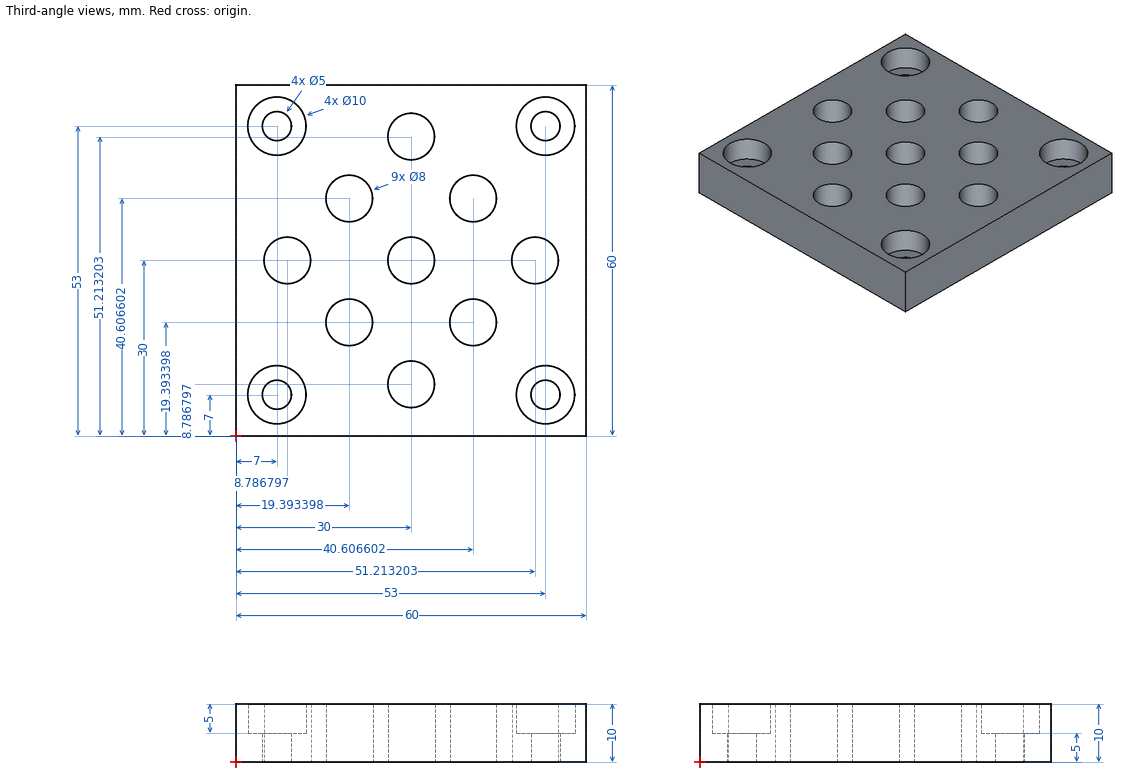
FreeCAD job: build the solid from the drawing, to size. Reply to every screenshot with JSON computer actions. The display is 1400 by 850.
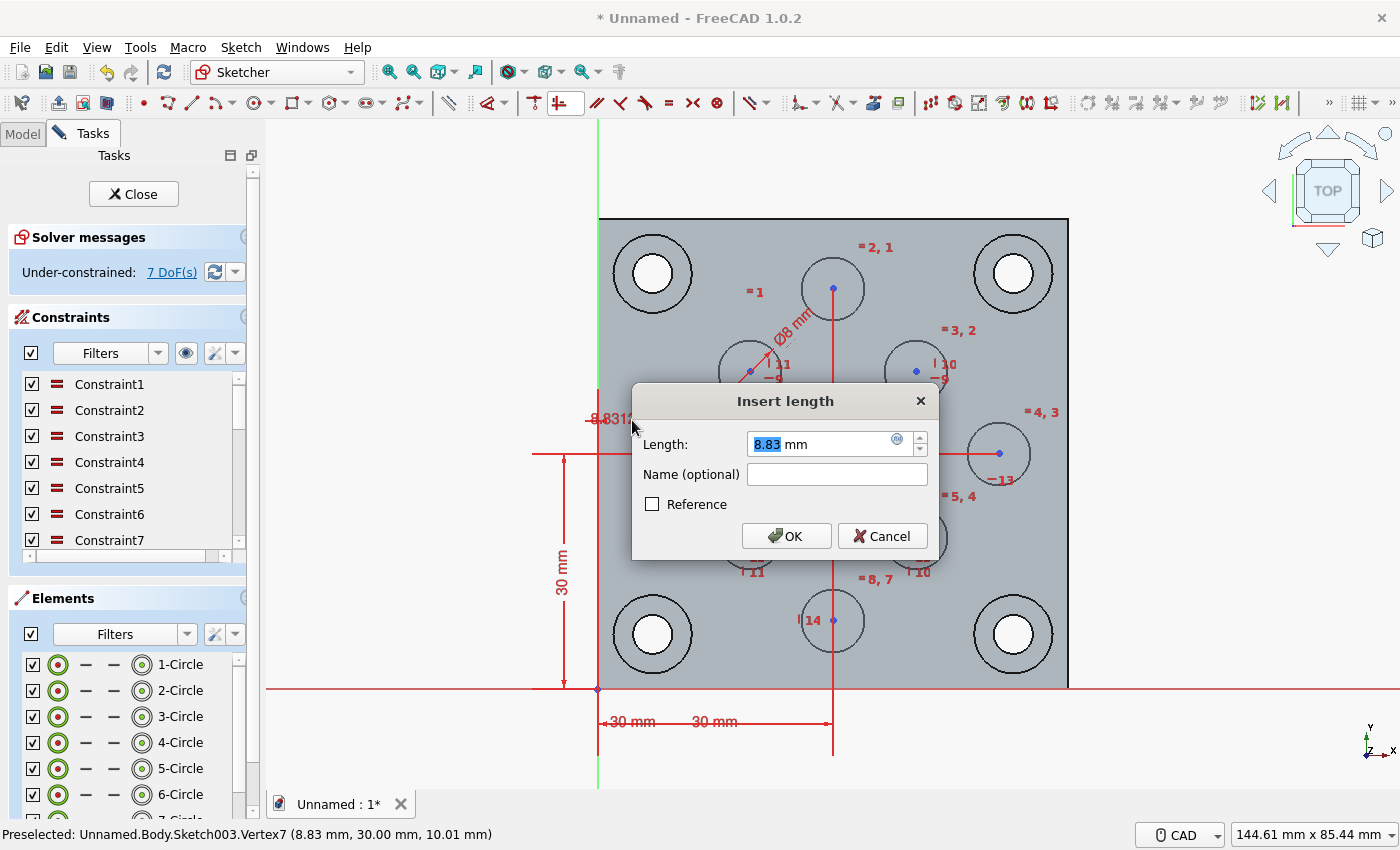
{"action": "type", "text": "8.786797"}
{"action": "key", "text": "Return"}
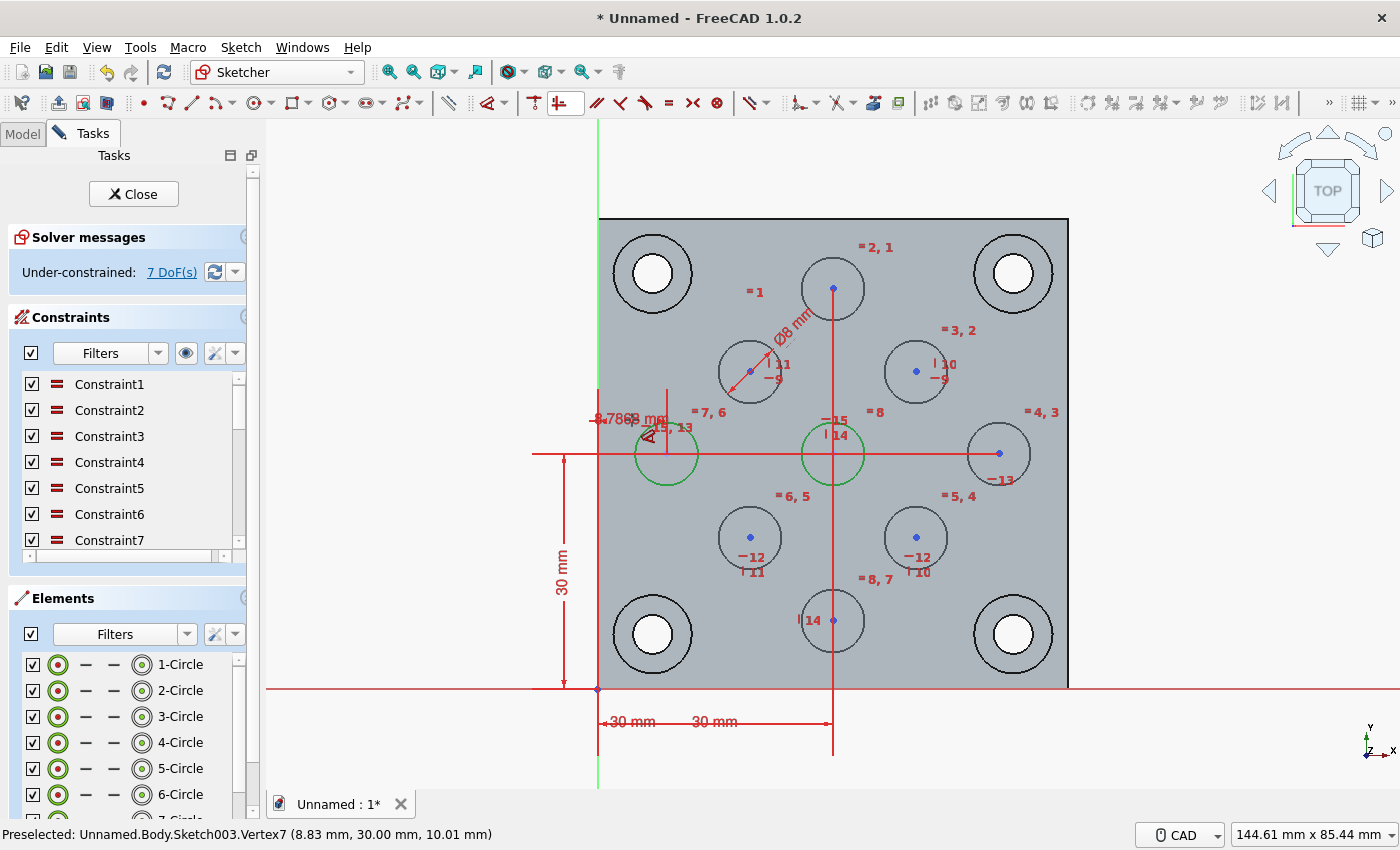
{"action": "left_click", "coordinate": [833, 621]}
{"action": "left_click", "coordinate": [564, 655]}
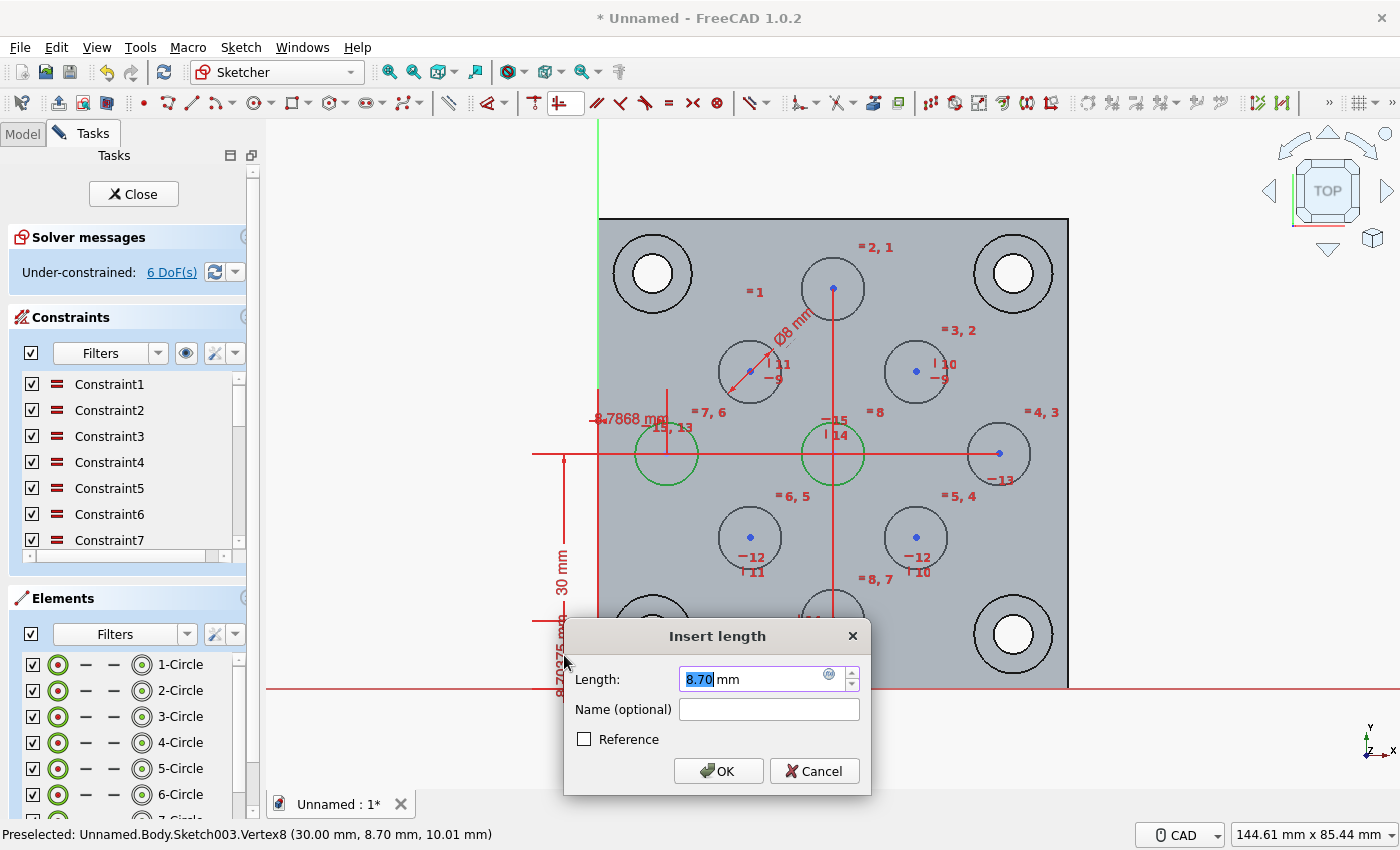
{"action": "type", "text": "8.786797"}
{"action": "key", "text": "Return"}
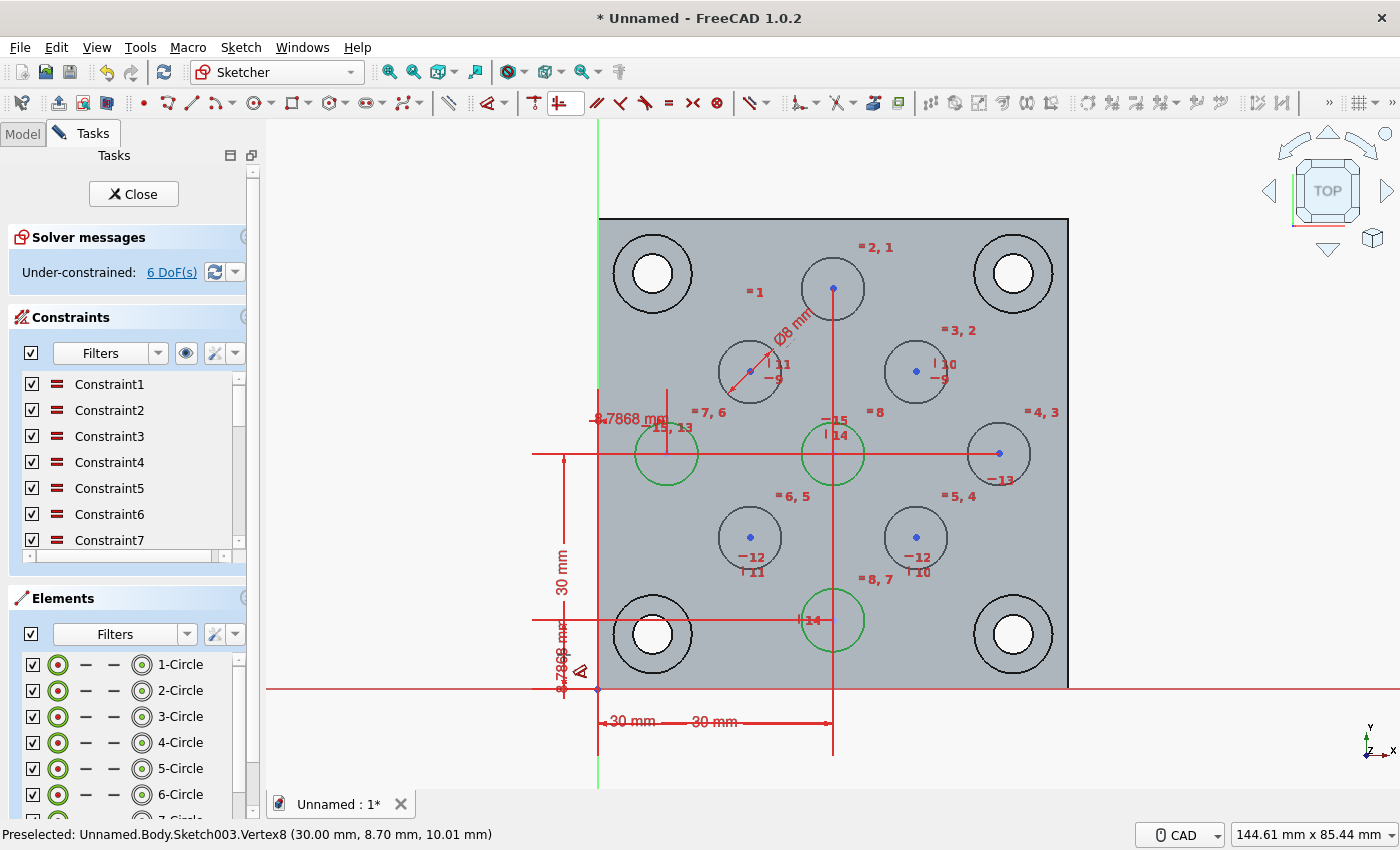
{"action": "left_click", "coordinate": [750, 372]}
{"action": "left_click", "coordinate": [674, 338]}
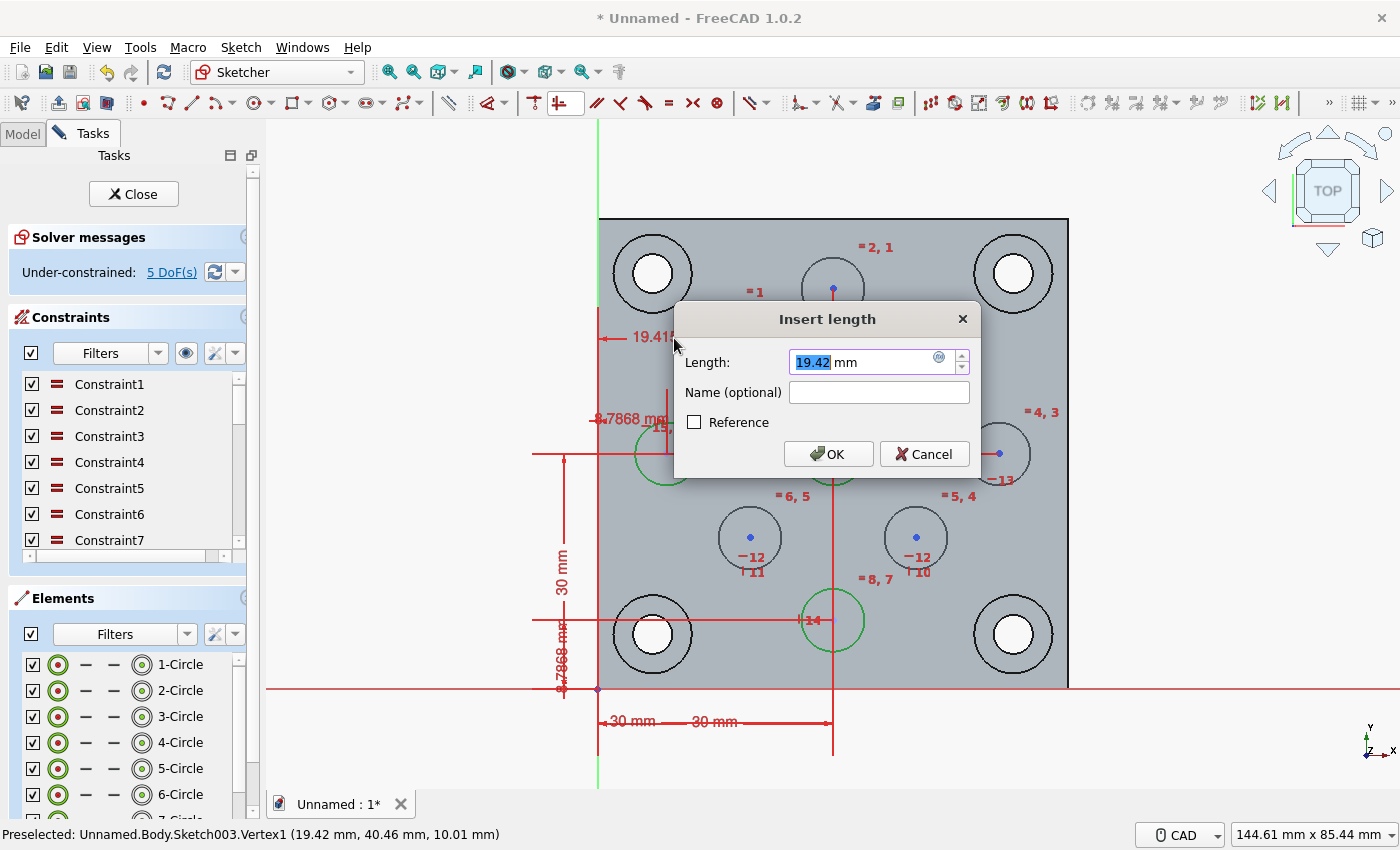
{"action": "type", "text": "19.393398"}
{"action": "key", "text": "Return"}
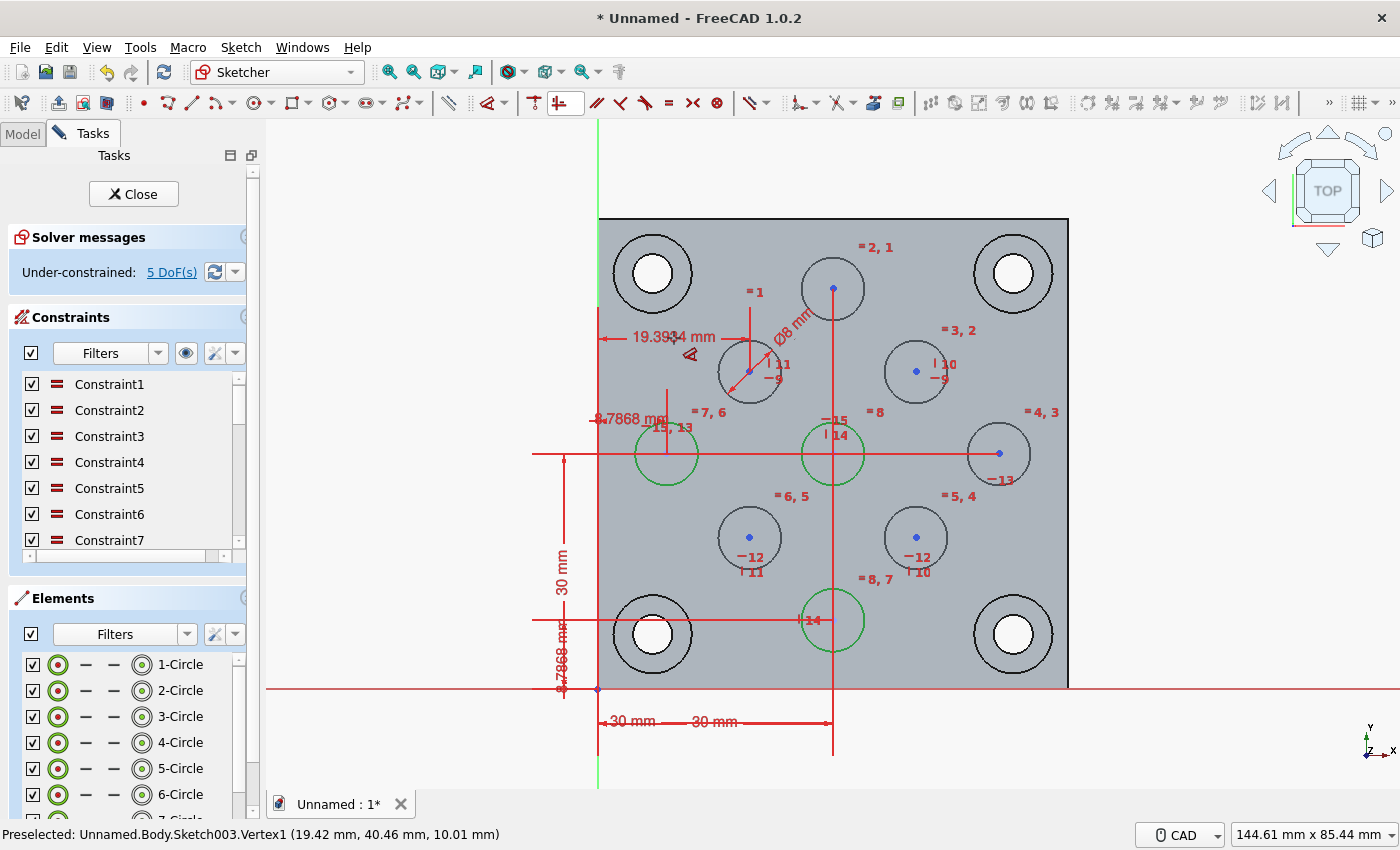
{"action": "left_click", "coordinate": [750, 372]}
{"action": "left_click", "coordinate": [564, 531]}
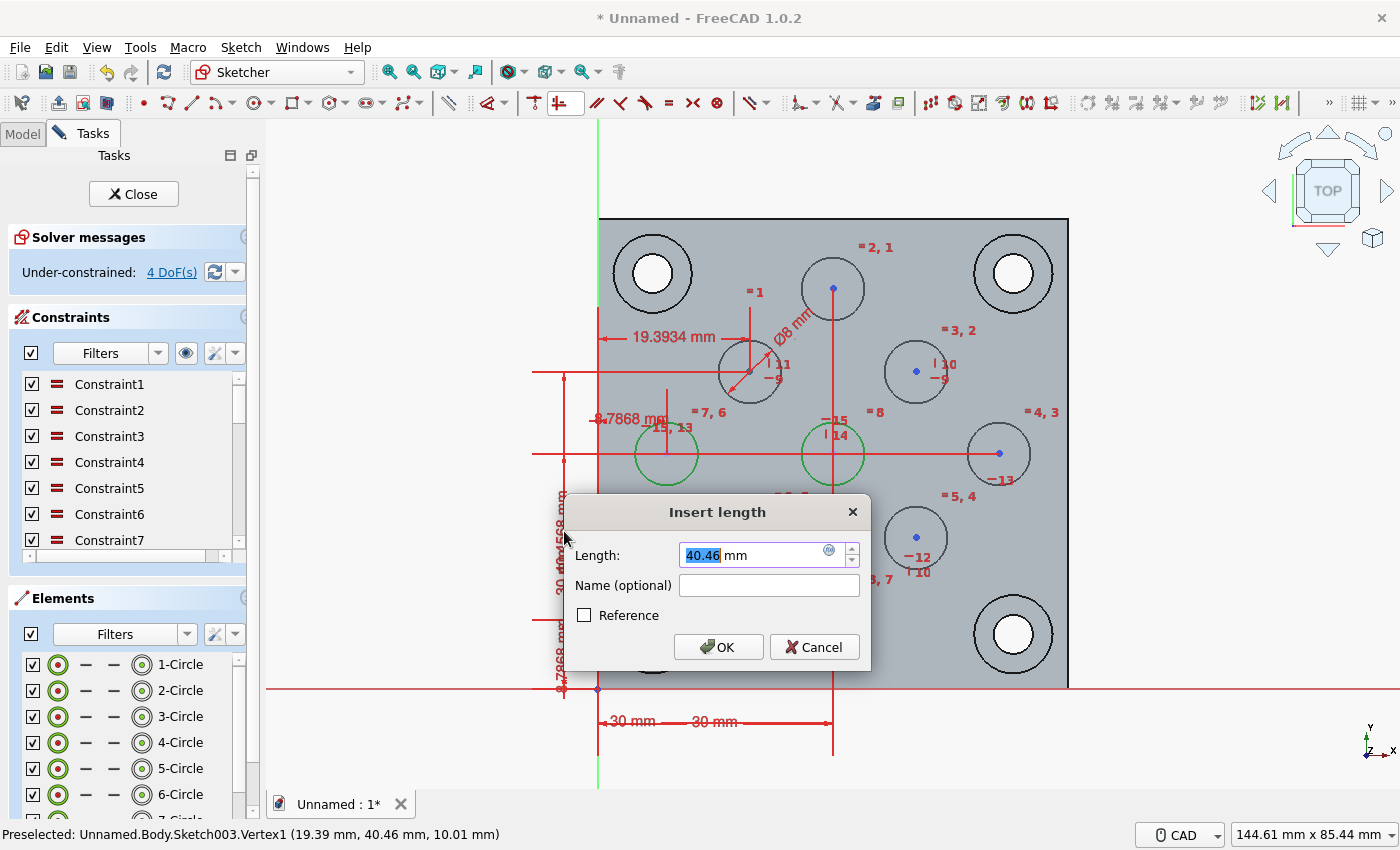
{"action": "type", "text": "40.606602"}
{"action": "key", "text": "Return"}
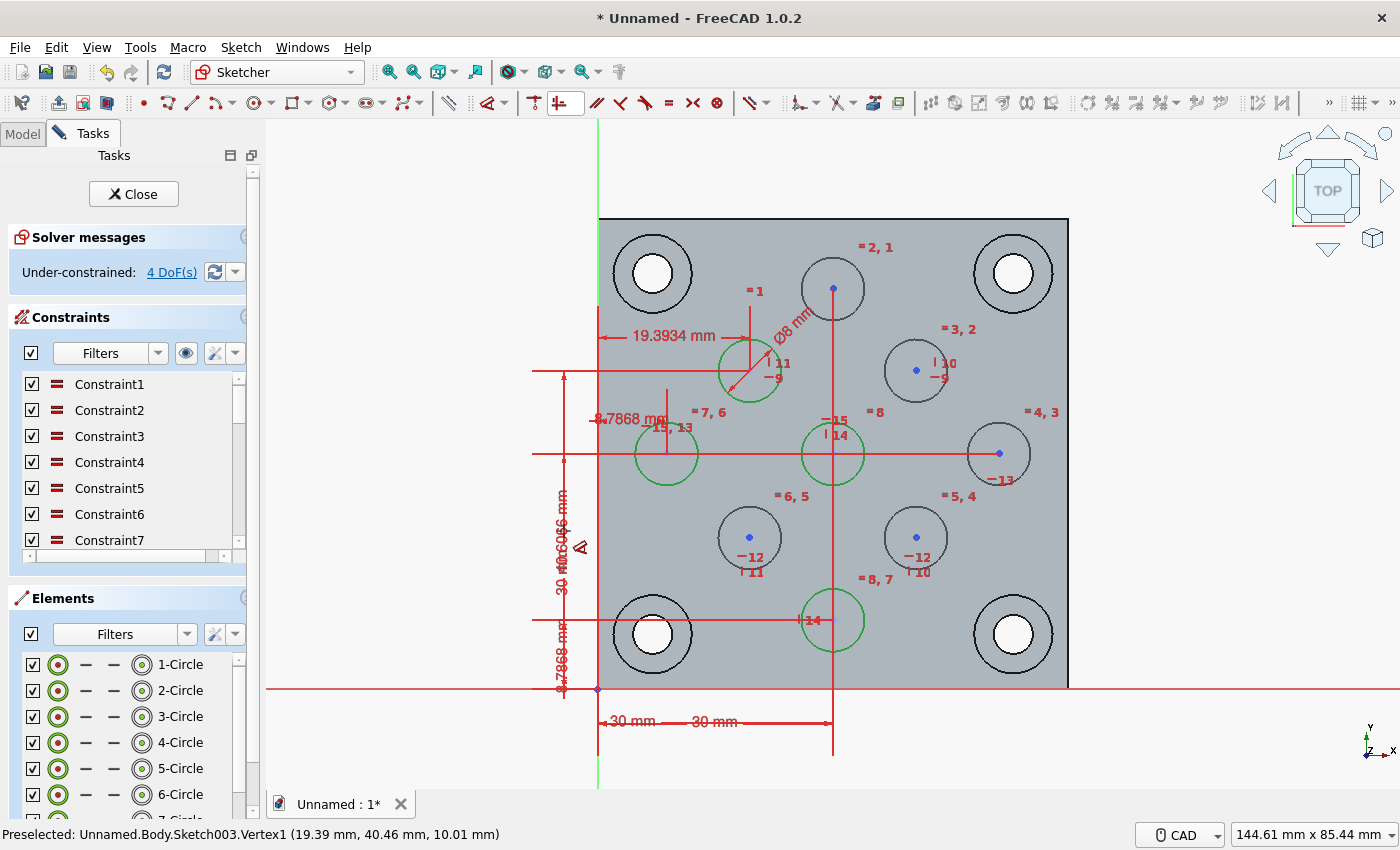
{"action": "left_click", "coordinate": [833, 289]}
{"action": "left_click", "coordinate": [564, 489]}